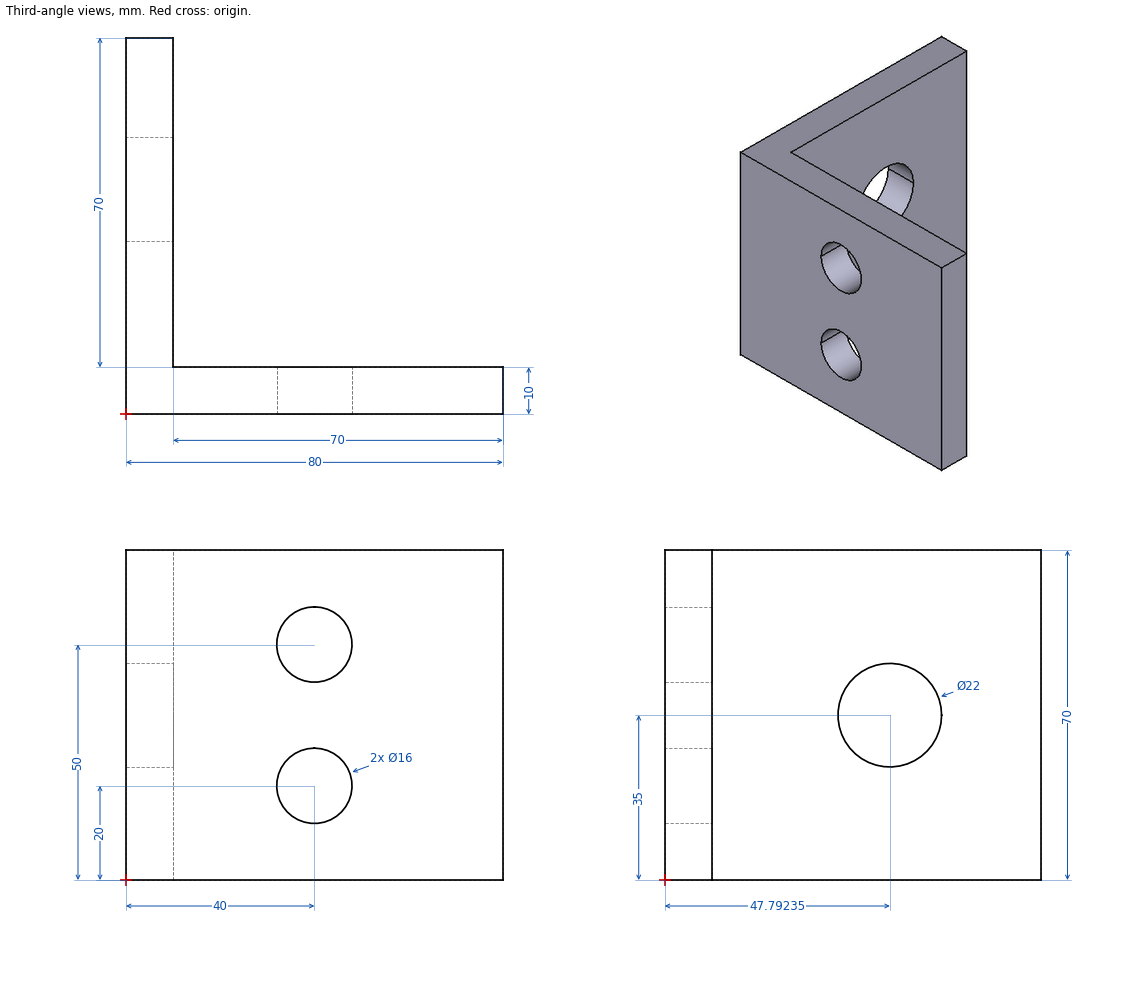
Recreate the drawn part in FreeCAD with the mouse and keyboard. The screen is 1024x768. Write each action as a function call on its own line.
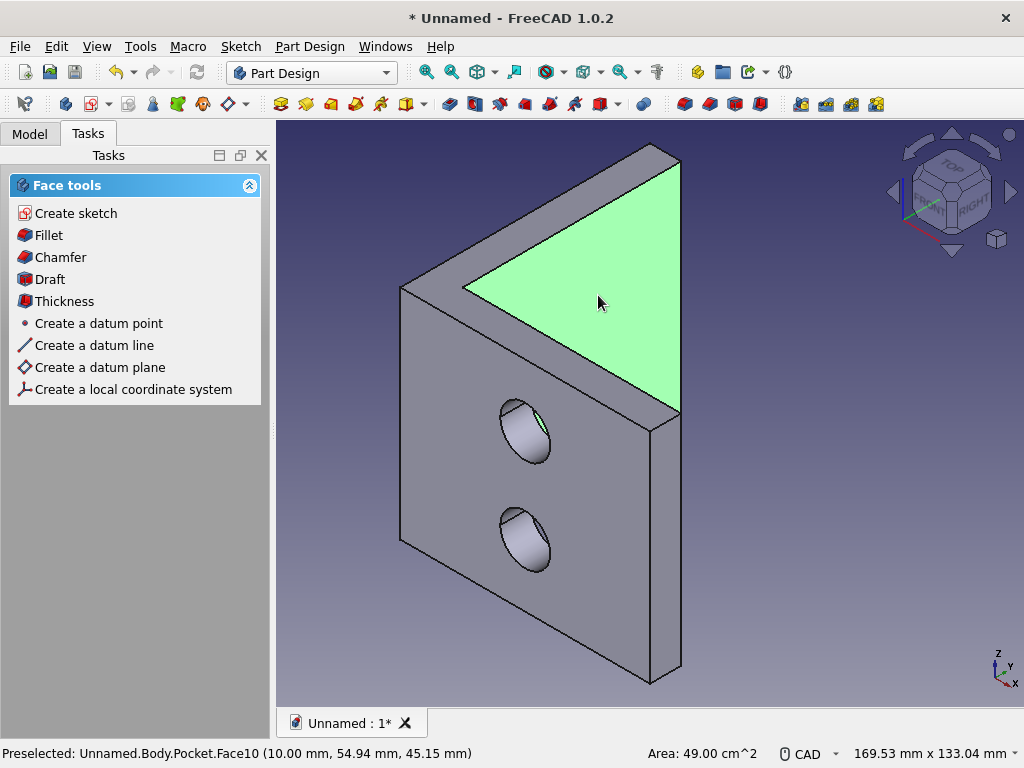
click(90, 104)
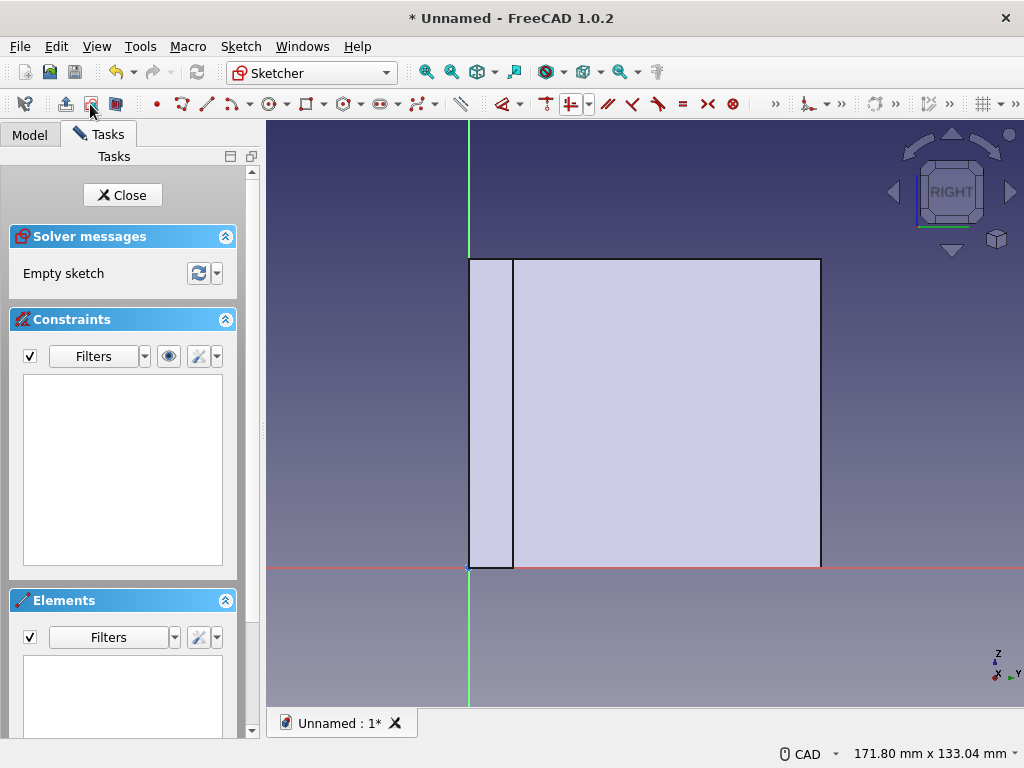
click(116, 104)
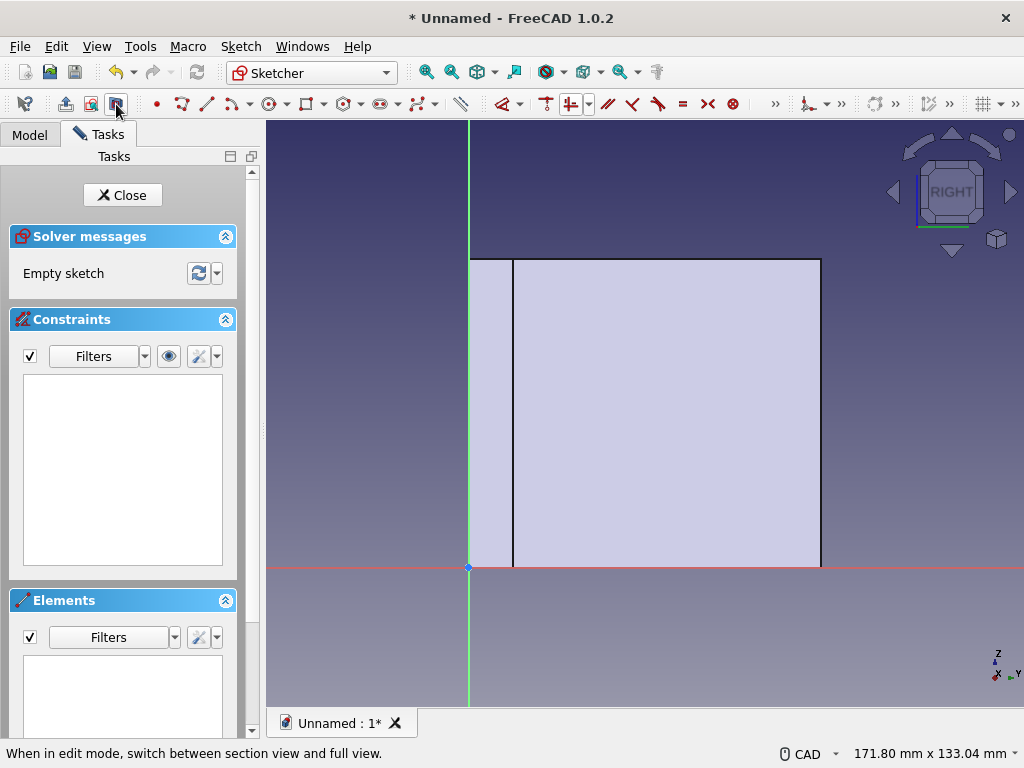
scroll(713, 414, up, 7)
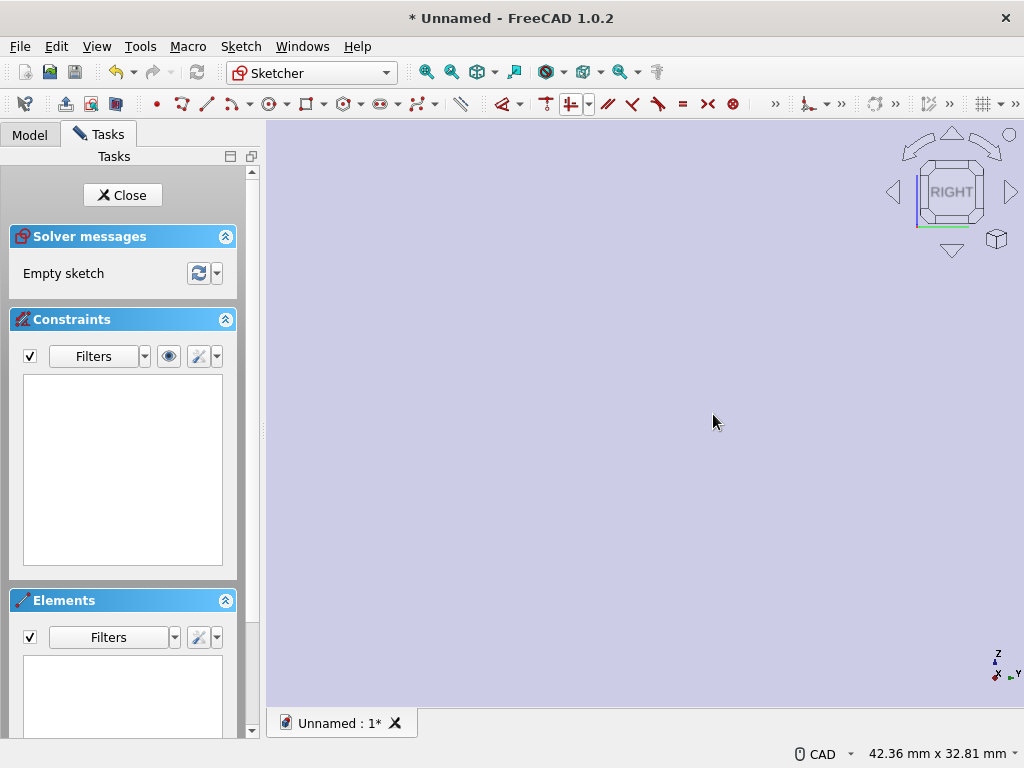
click(268, 104)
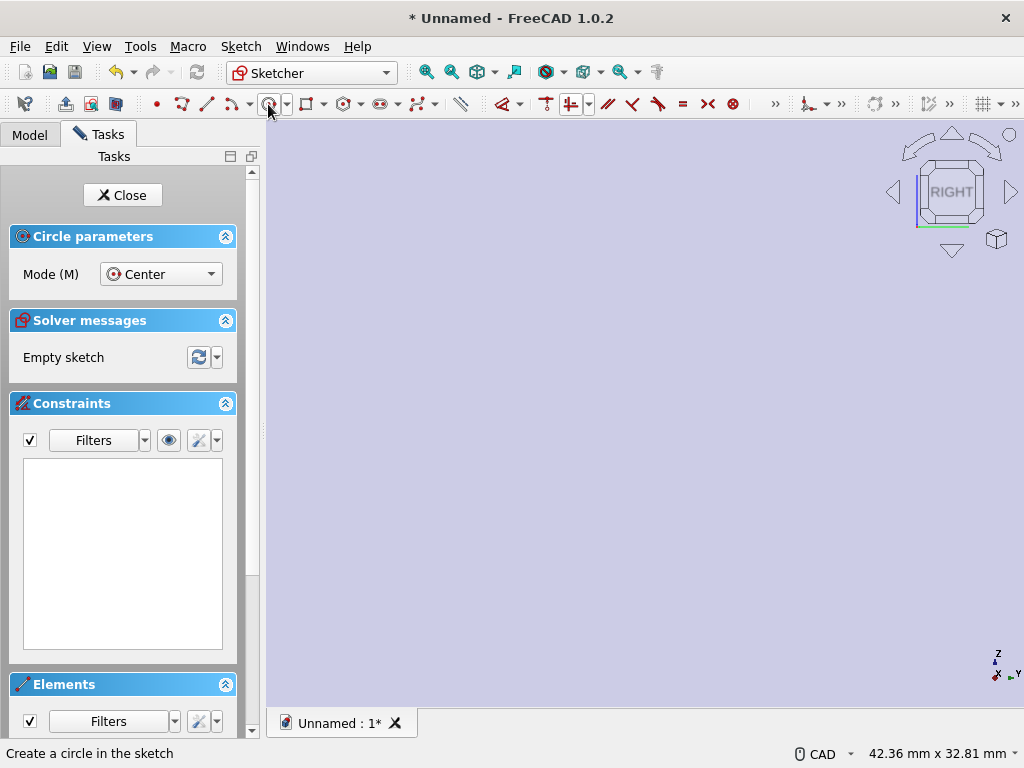
click(575, 410)
click(714, 271)
key(Escape)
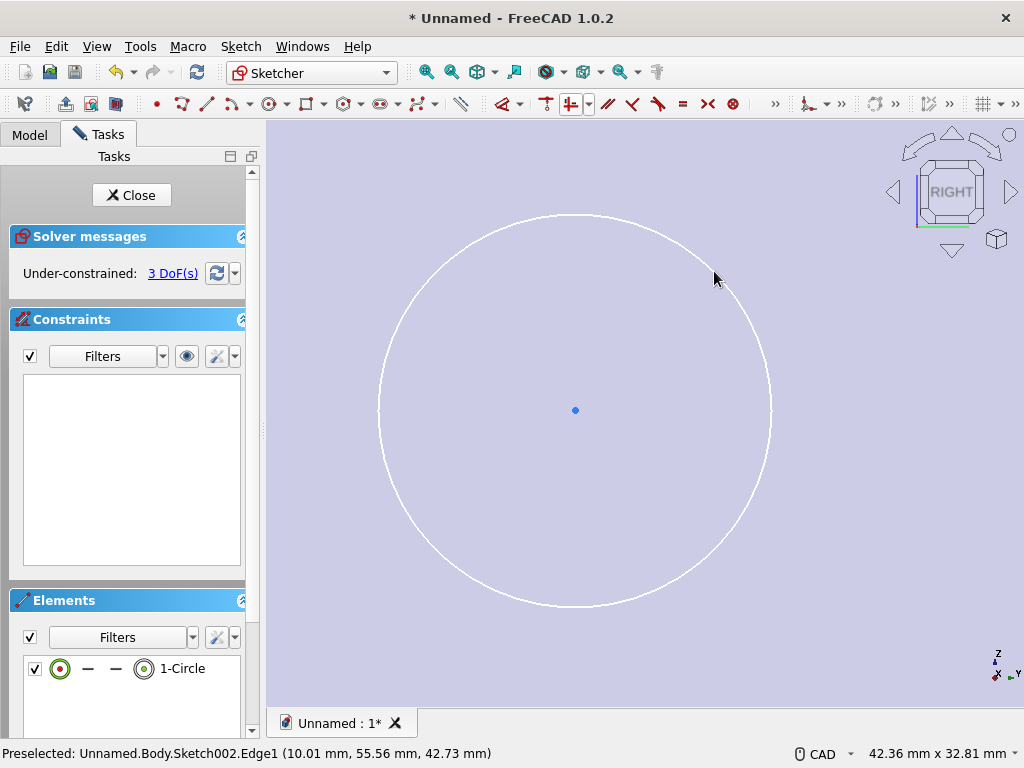
key(d)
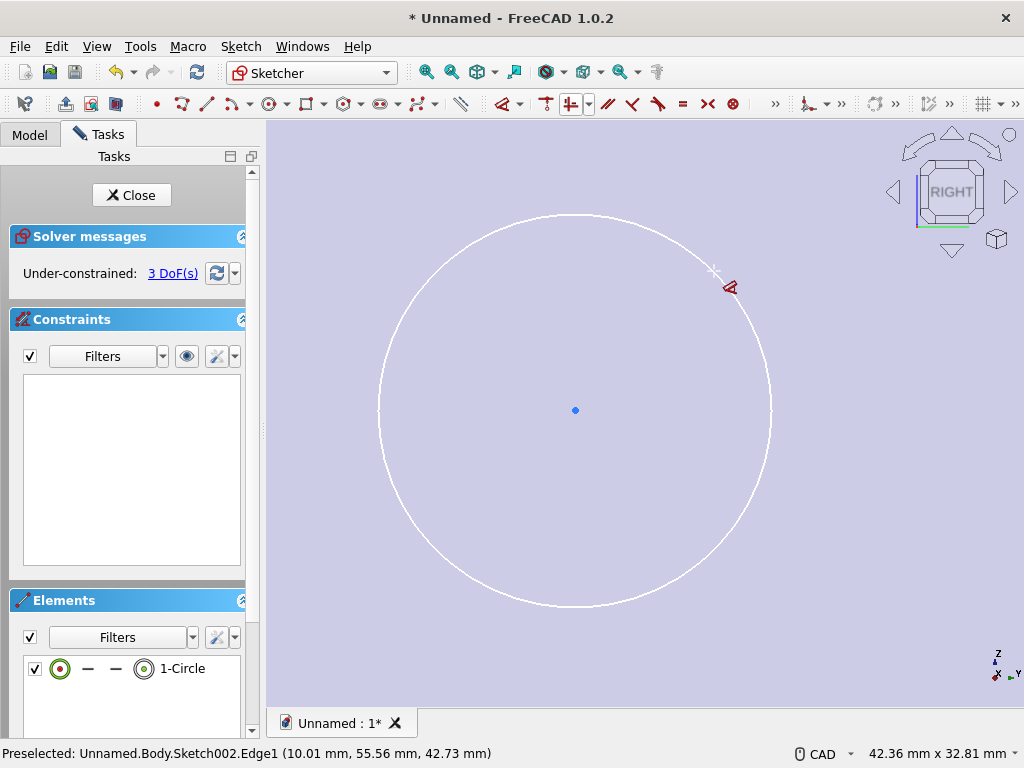
click(714, 272)
click(737, 249)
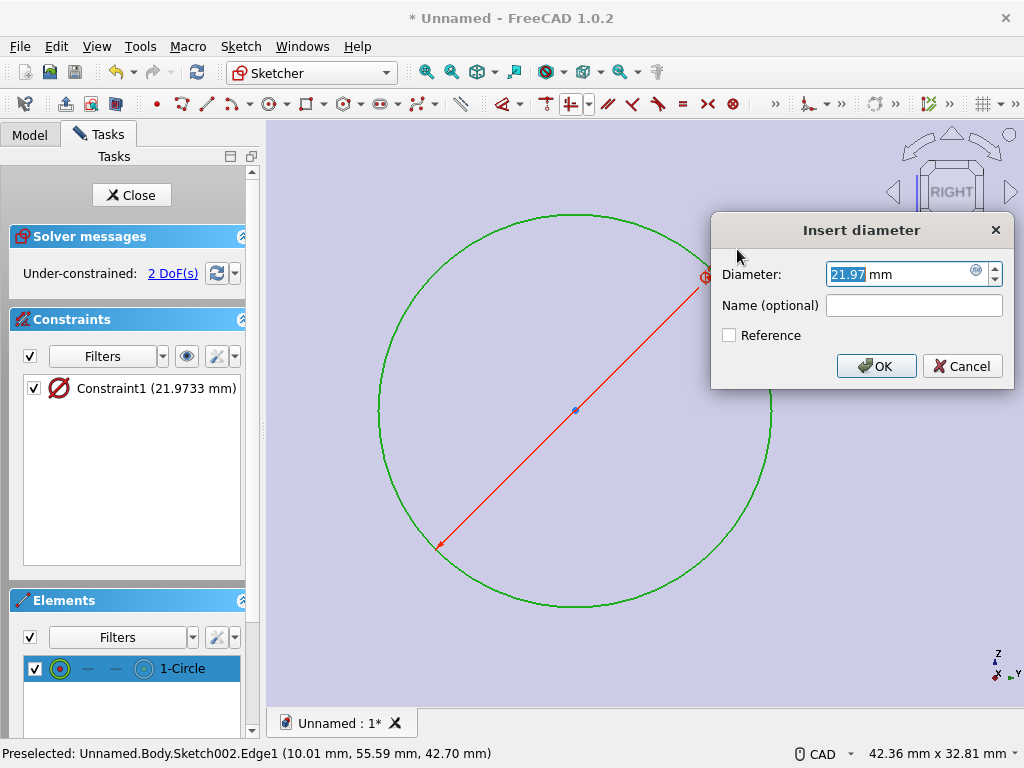
text(22)
key(Return)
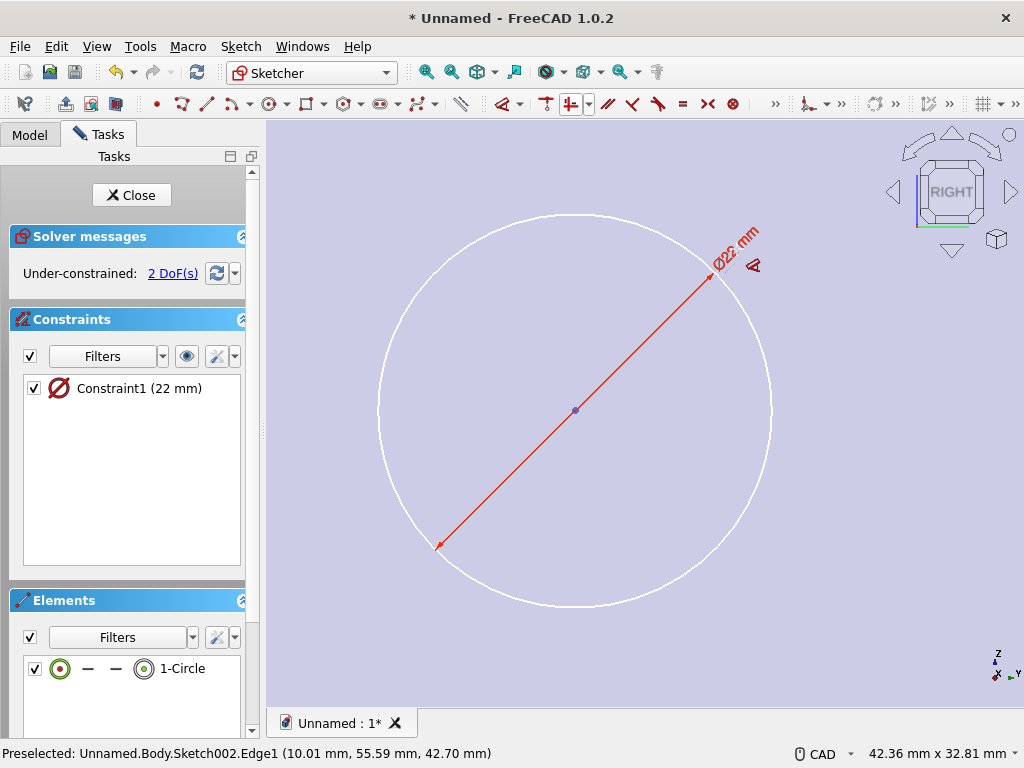
click(575, 411)
click(609, 545)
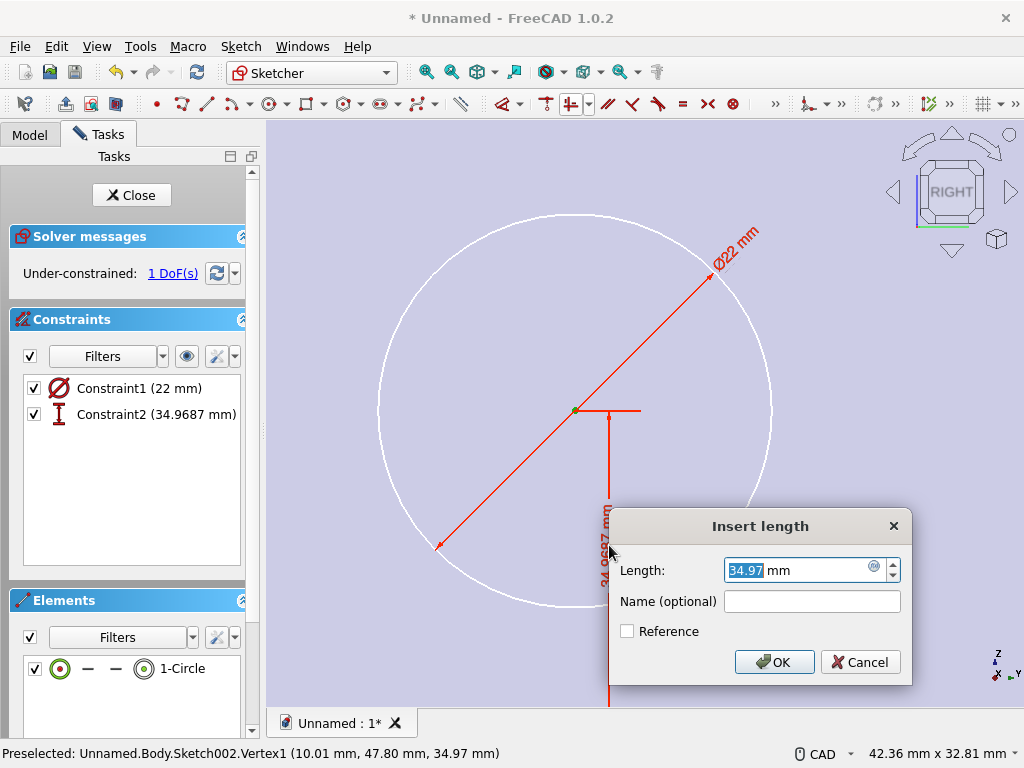
text(35)
key(Return)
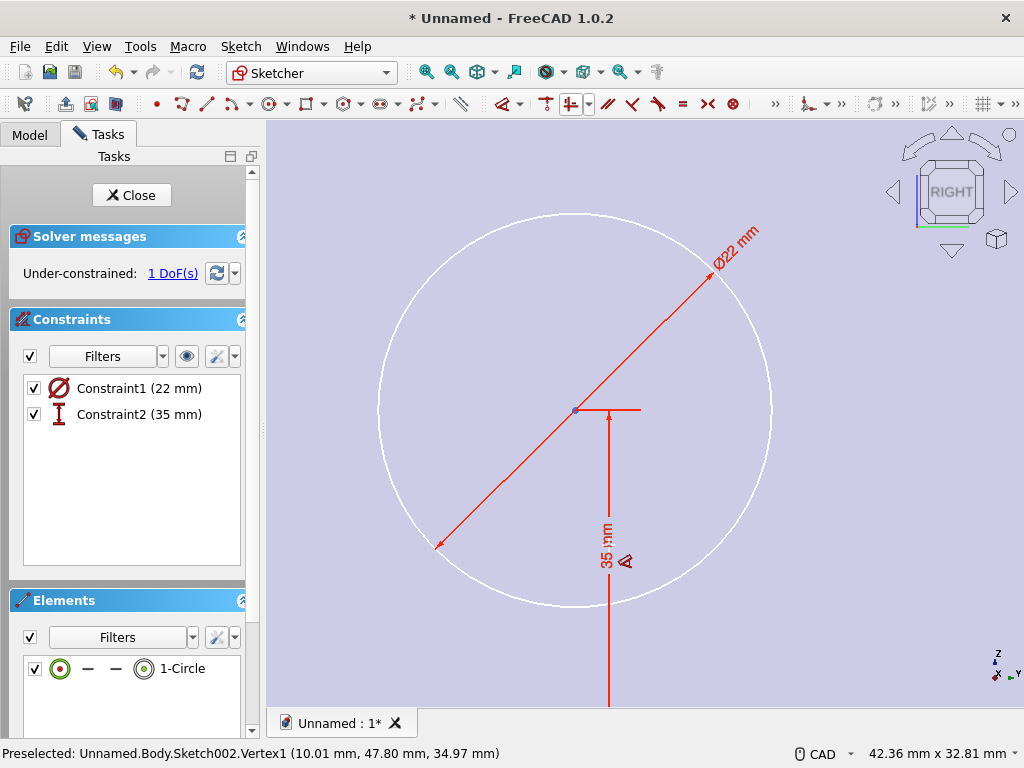
click(575, 410)
click(435, 376)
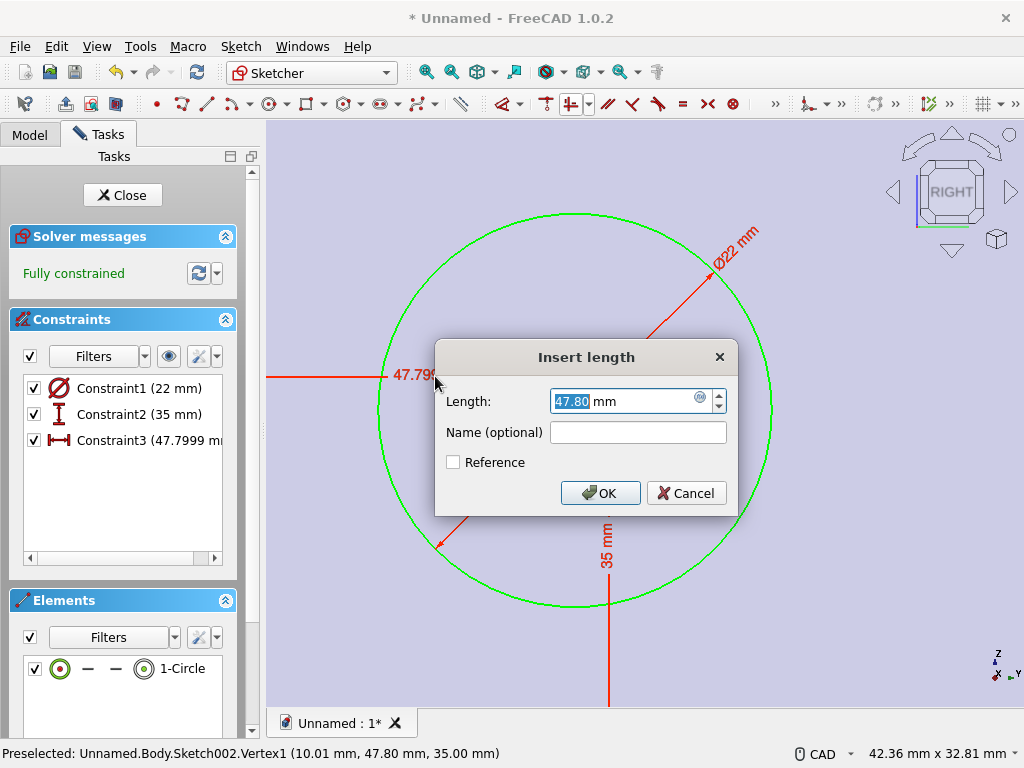
text(47.79235)
key(Return)
key(Escape)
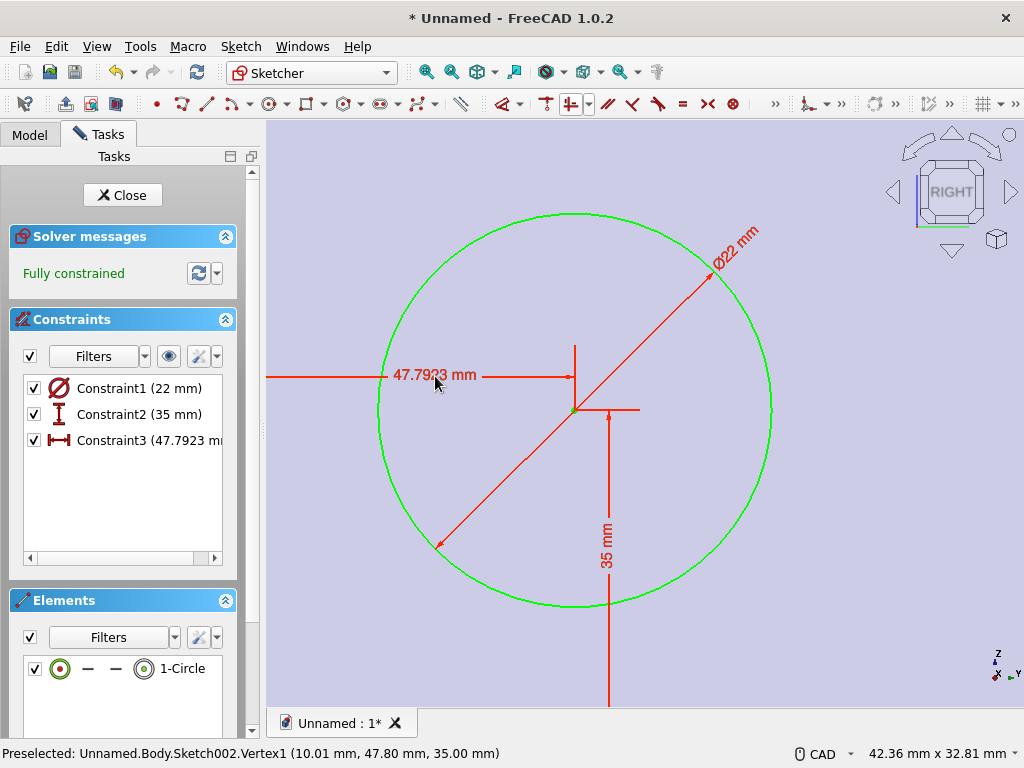
click(123, 195)